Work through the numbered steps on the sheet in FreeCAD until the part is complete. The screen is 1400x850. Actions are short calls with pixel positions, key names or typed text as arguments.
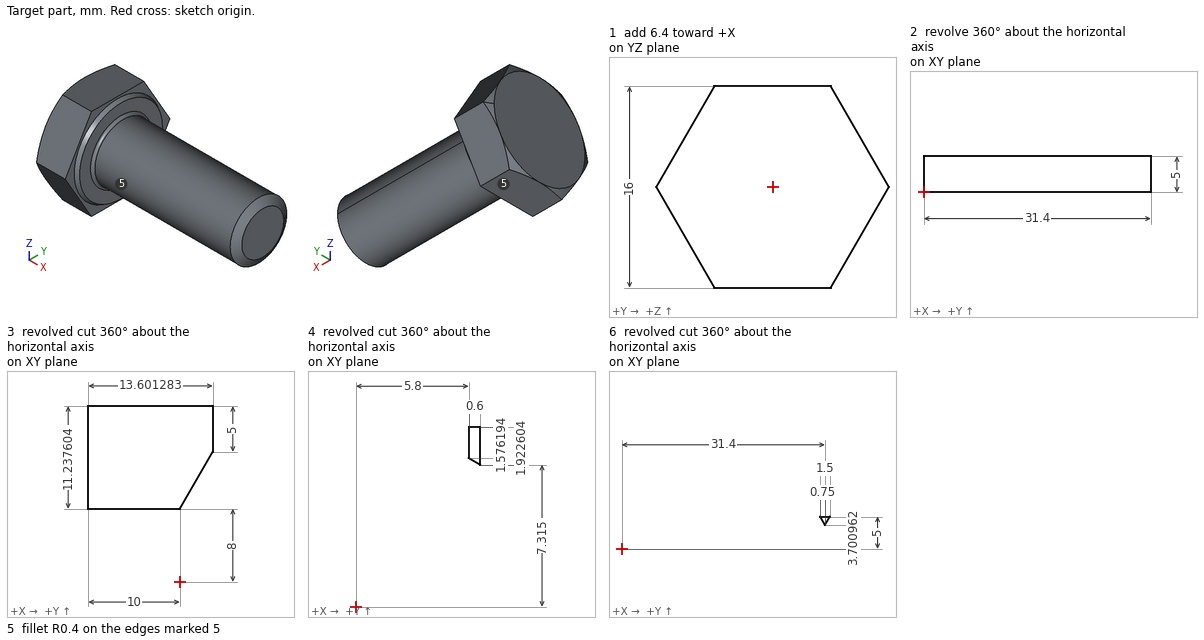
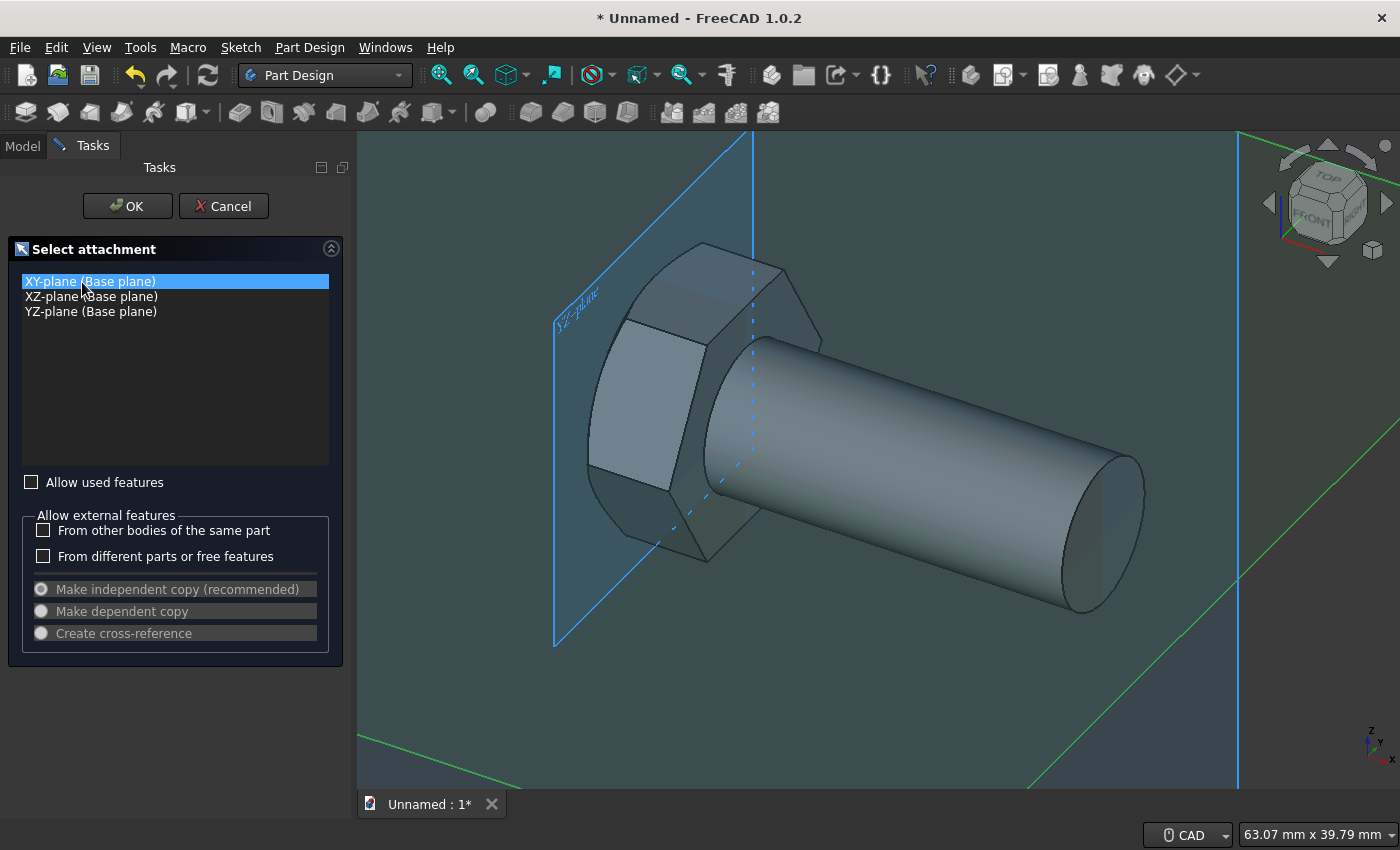
click(128, 206)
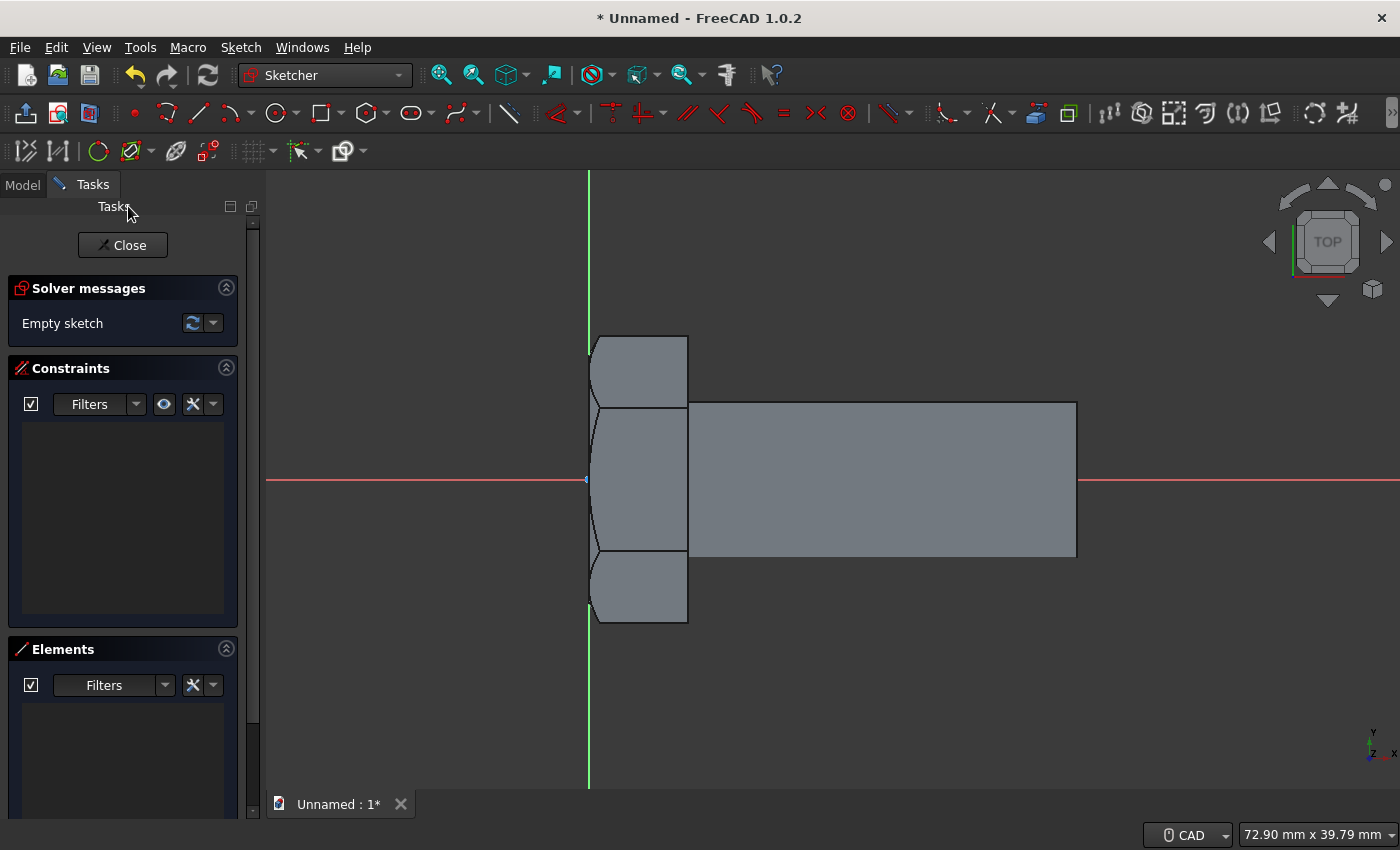
click(90, 114)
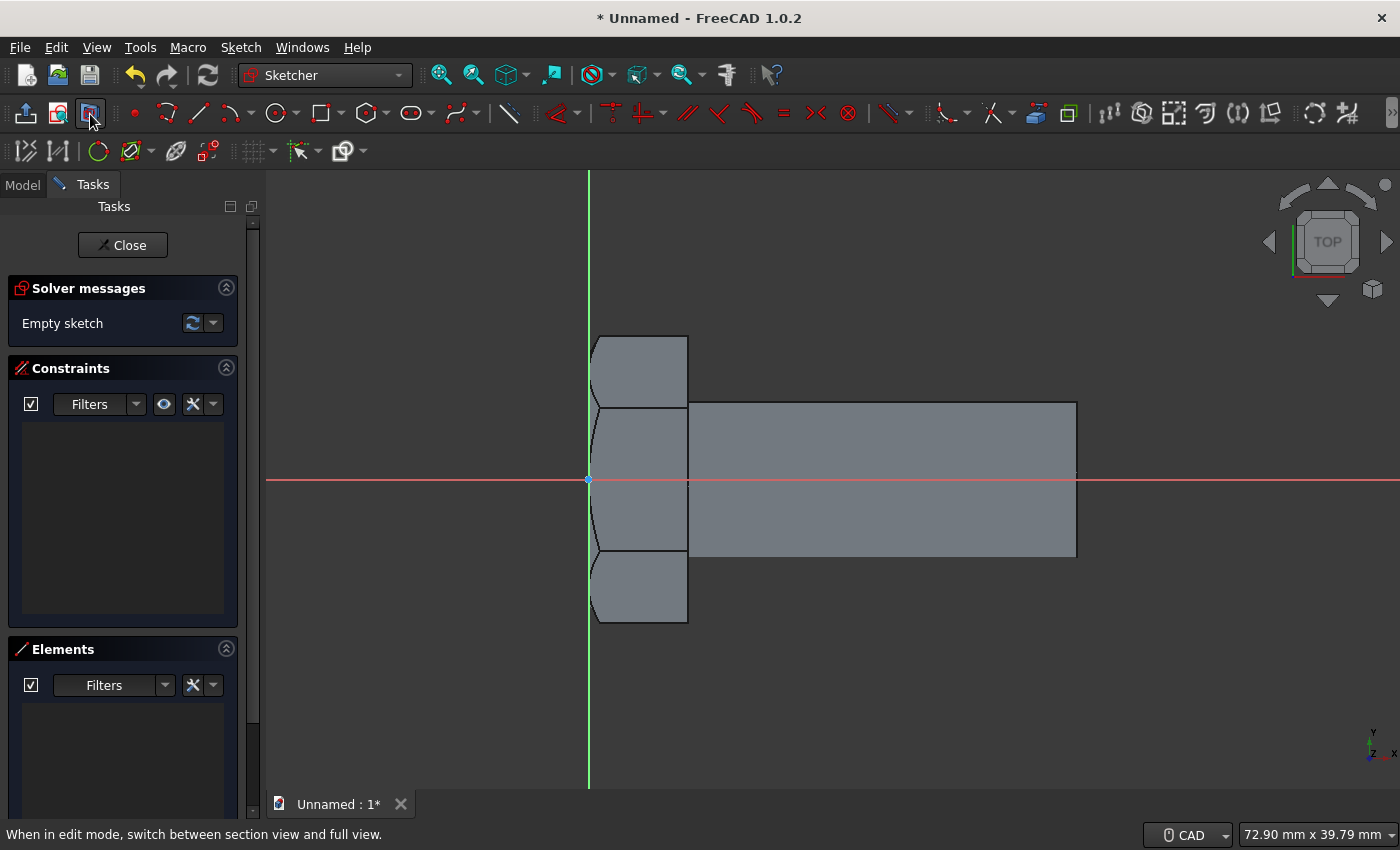
scroll(677, 340, up, 13)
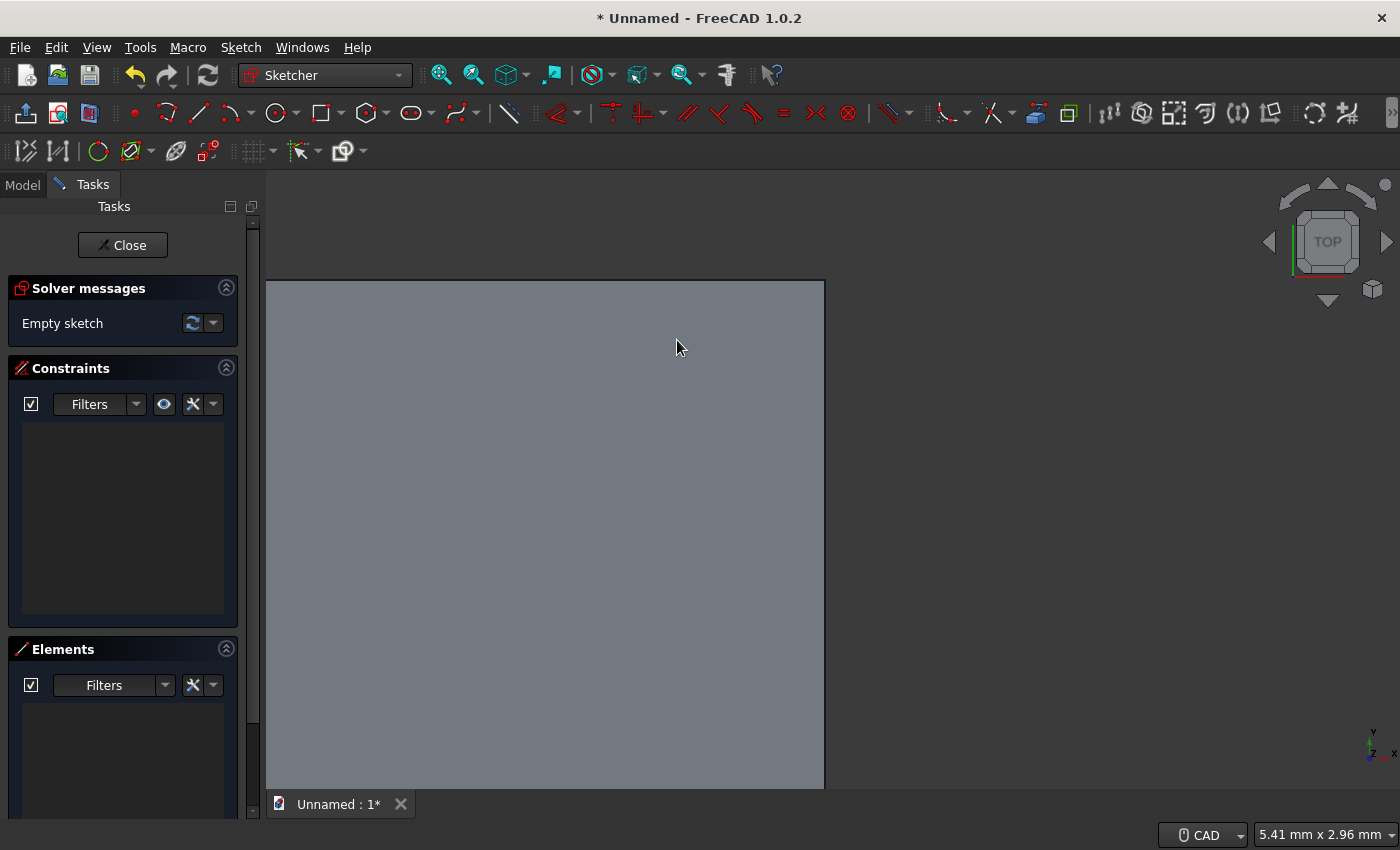
click(168, 114)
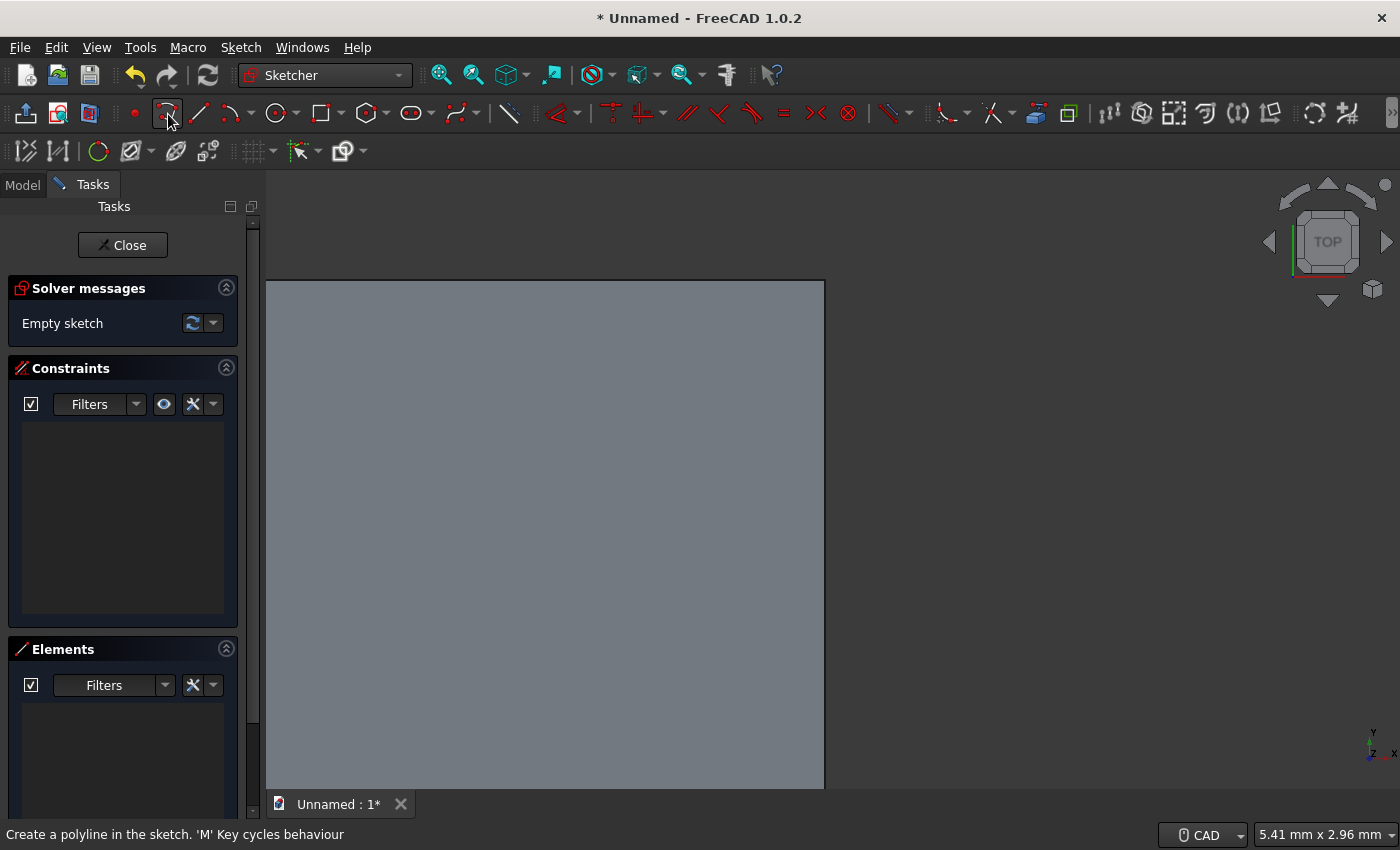
click(699, 610)
click(825, 683)
click(825, 280)
click(699, 280)
click(699, 611)
key(Escape)
key(Escape)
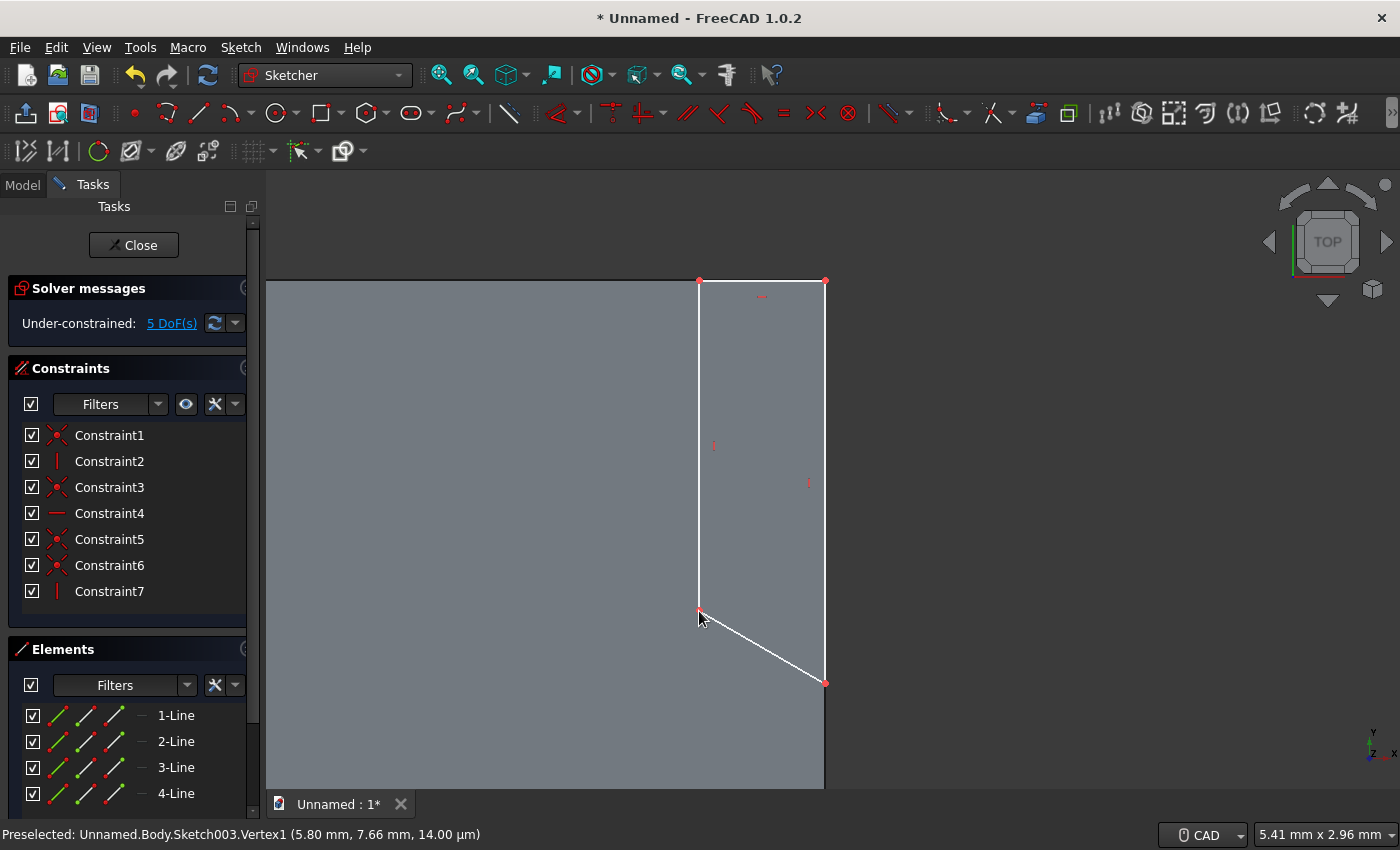
click(556, 114)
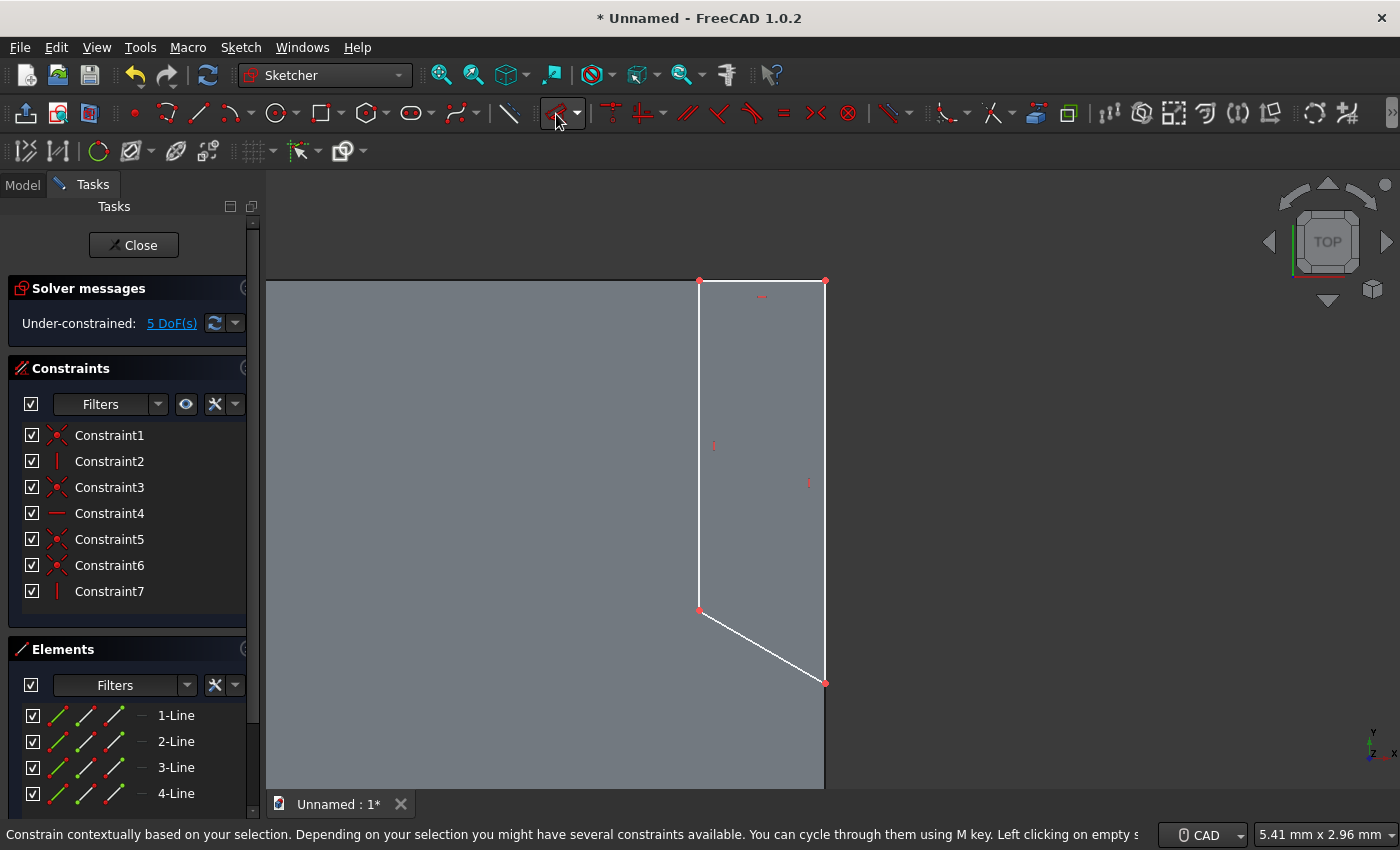
click(787, 281)
click(762, 247)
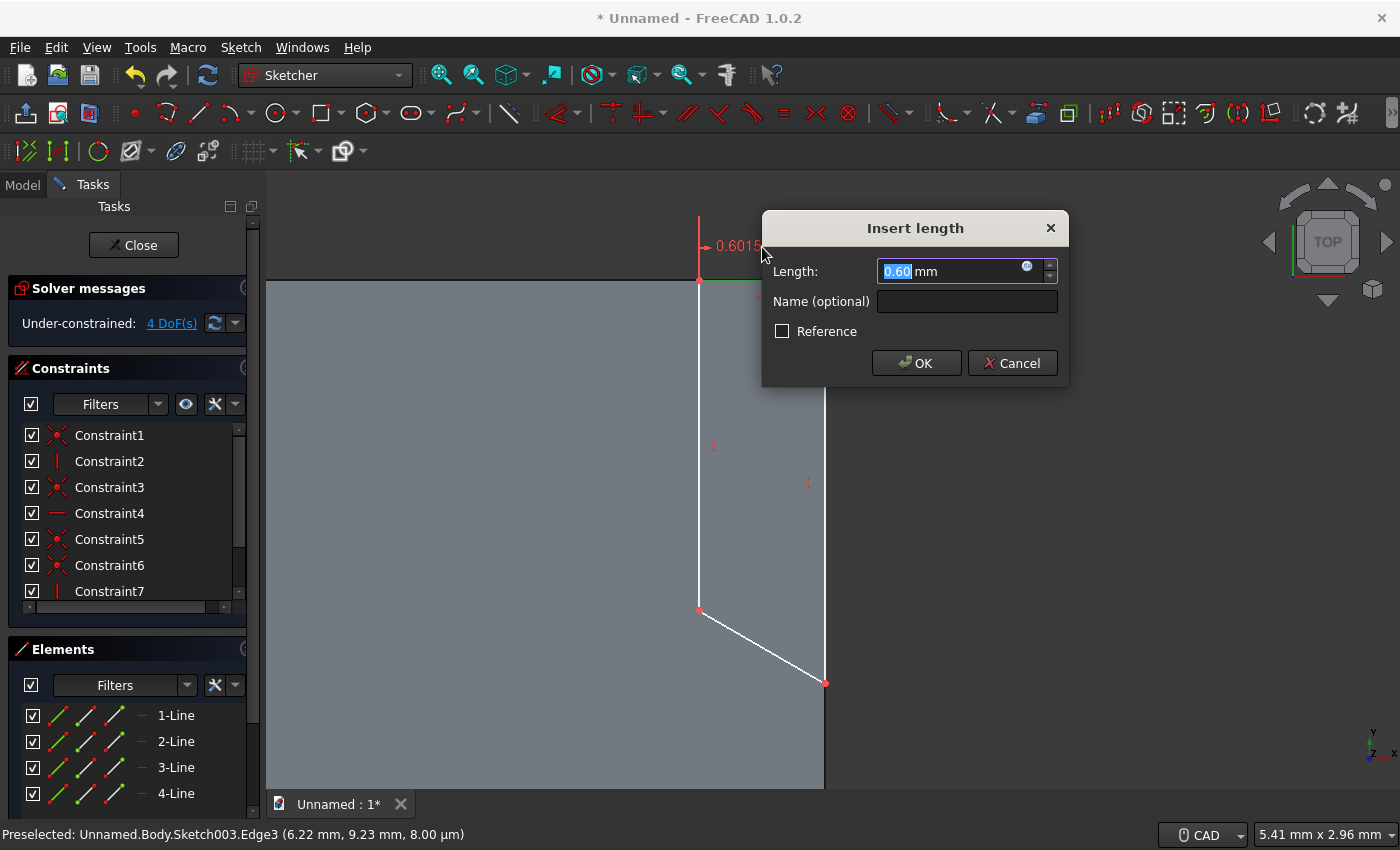
text(0.6)
key(Return)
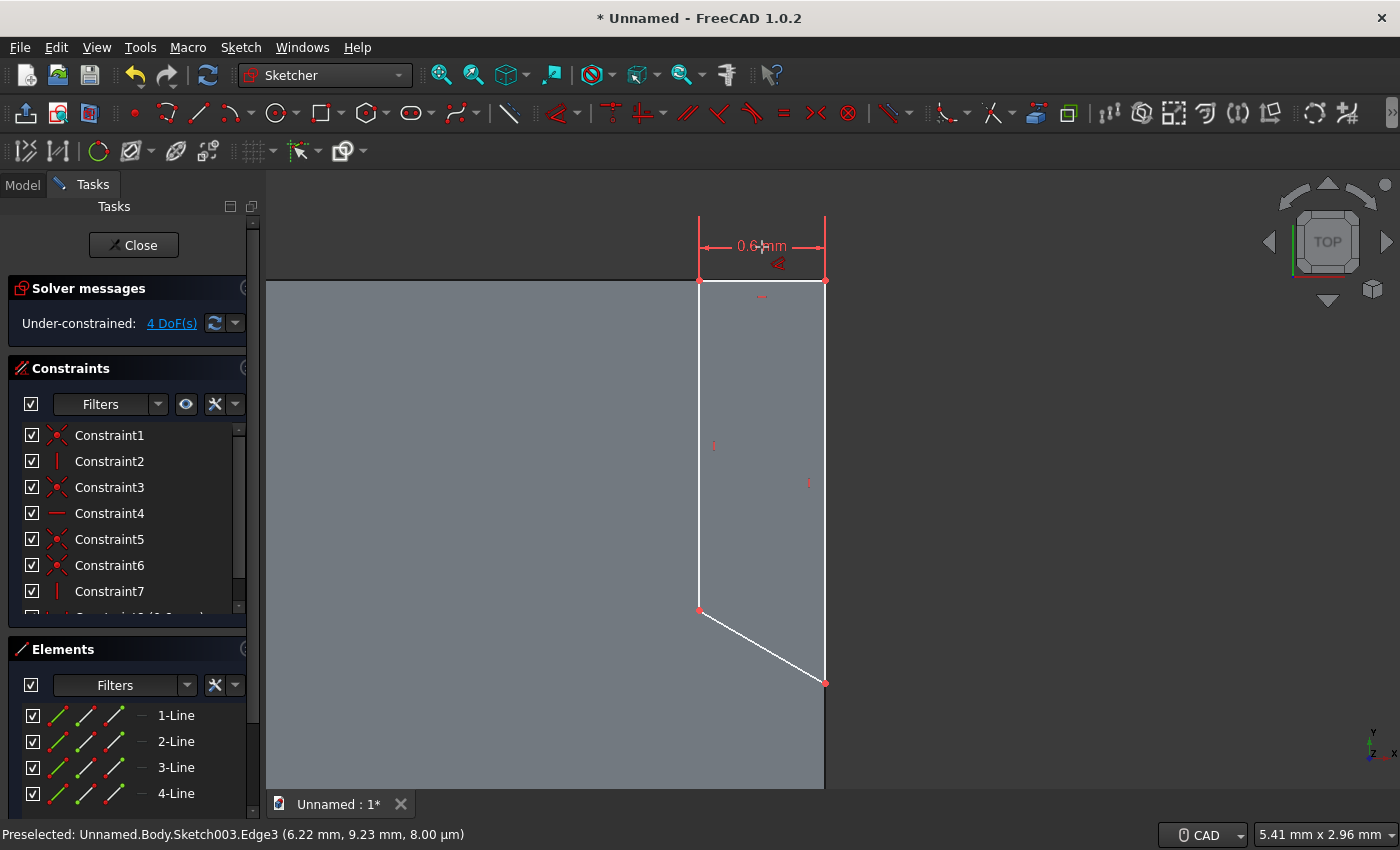
click(699, 611)
click(497, 577)